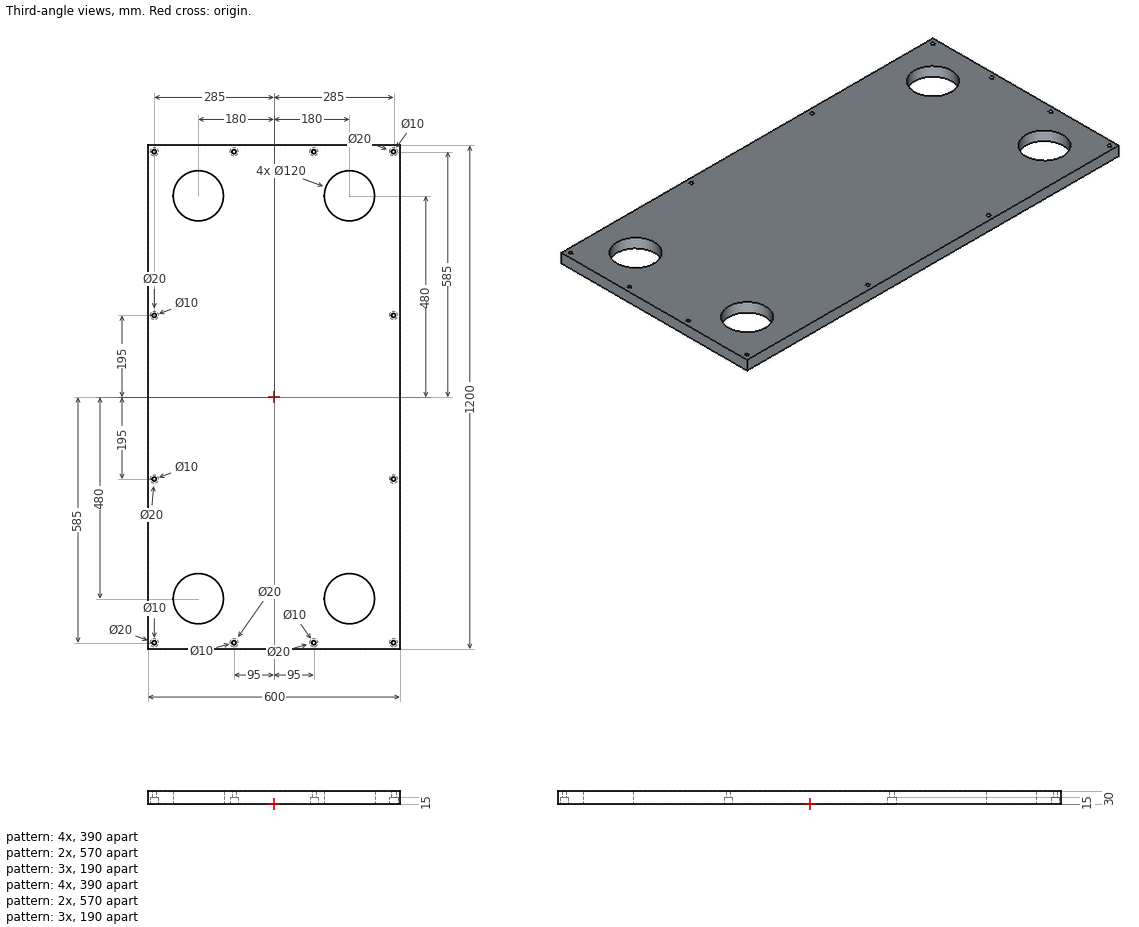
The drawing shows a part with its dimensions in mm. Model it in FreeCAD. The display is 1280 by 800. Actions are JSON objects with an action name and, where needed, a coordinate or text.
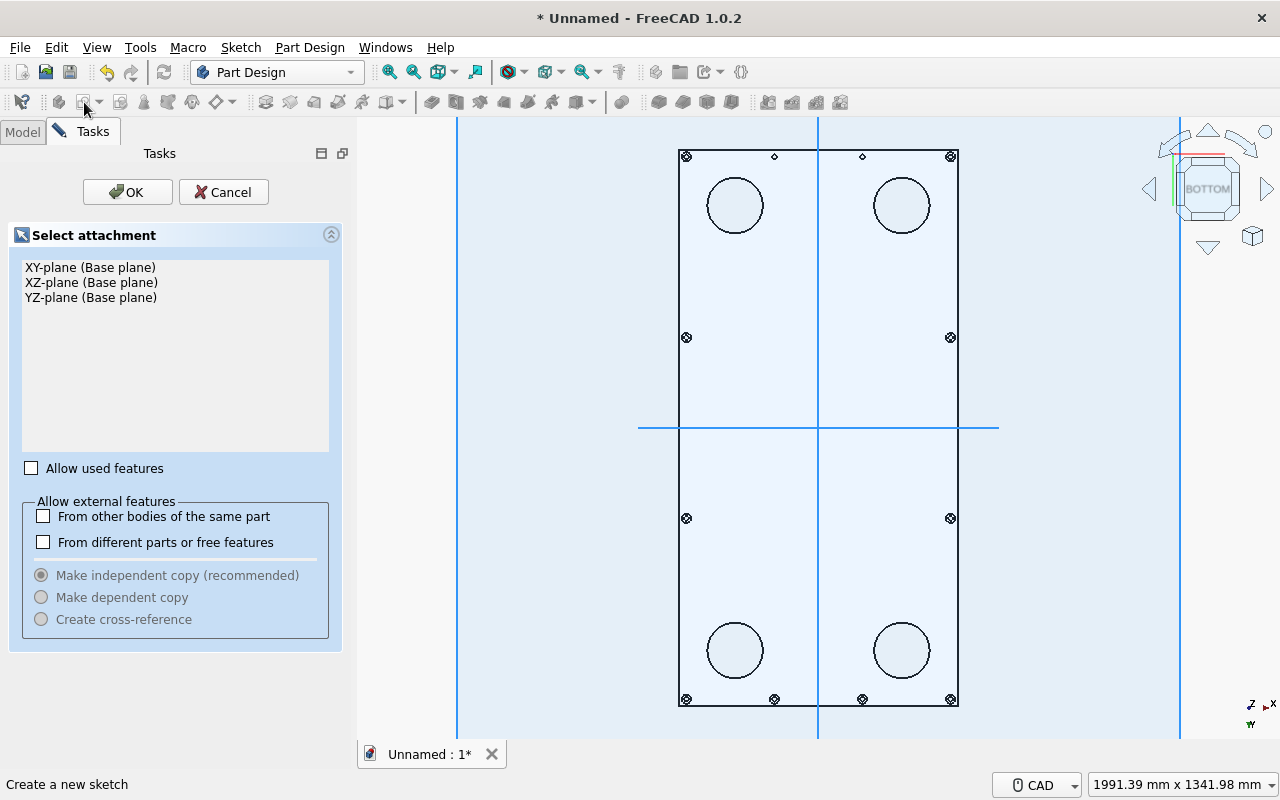
{"action": "left_click", "coordinate": [82, 268]}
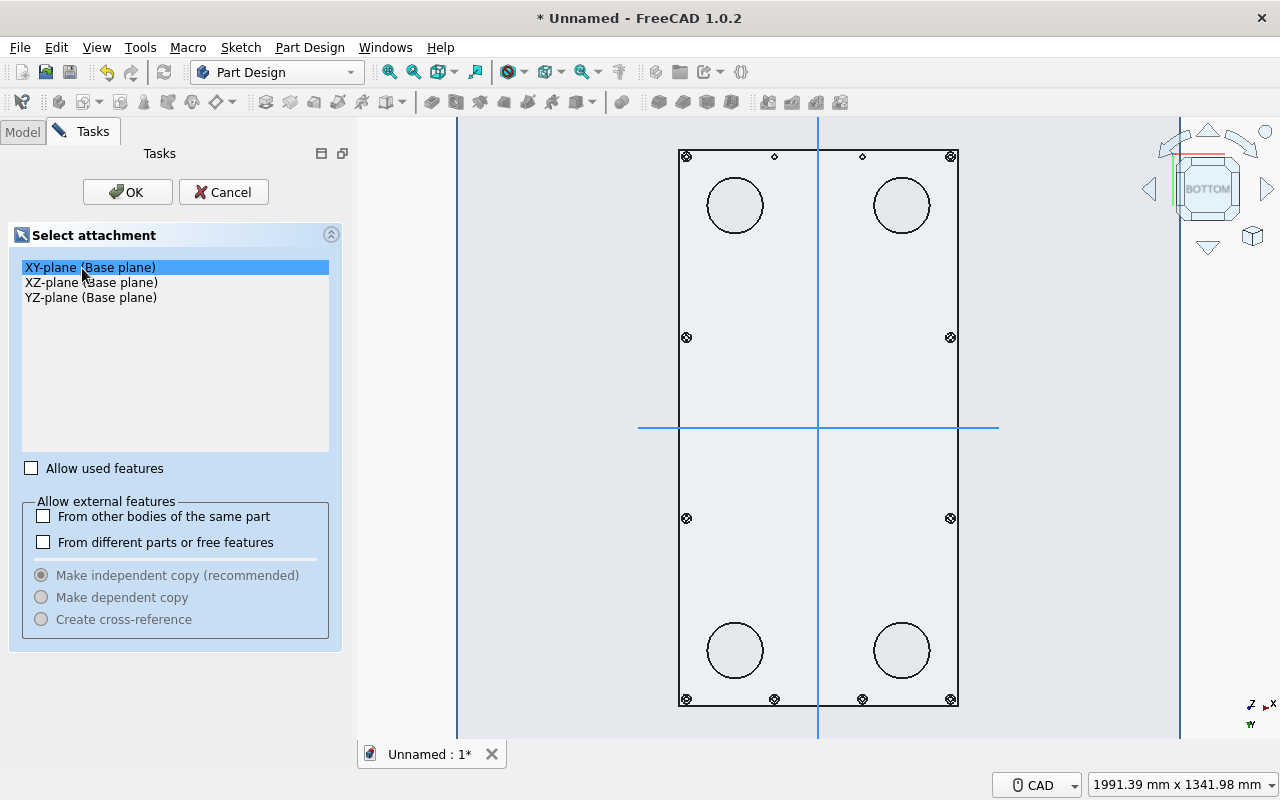
{"action": "left_click", "coordinate": [128, 192]}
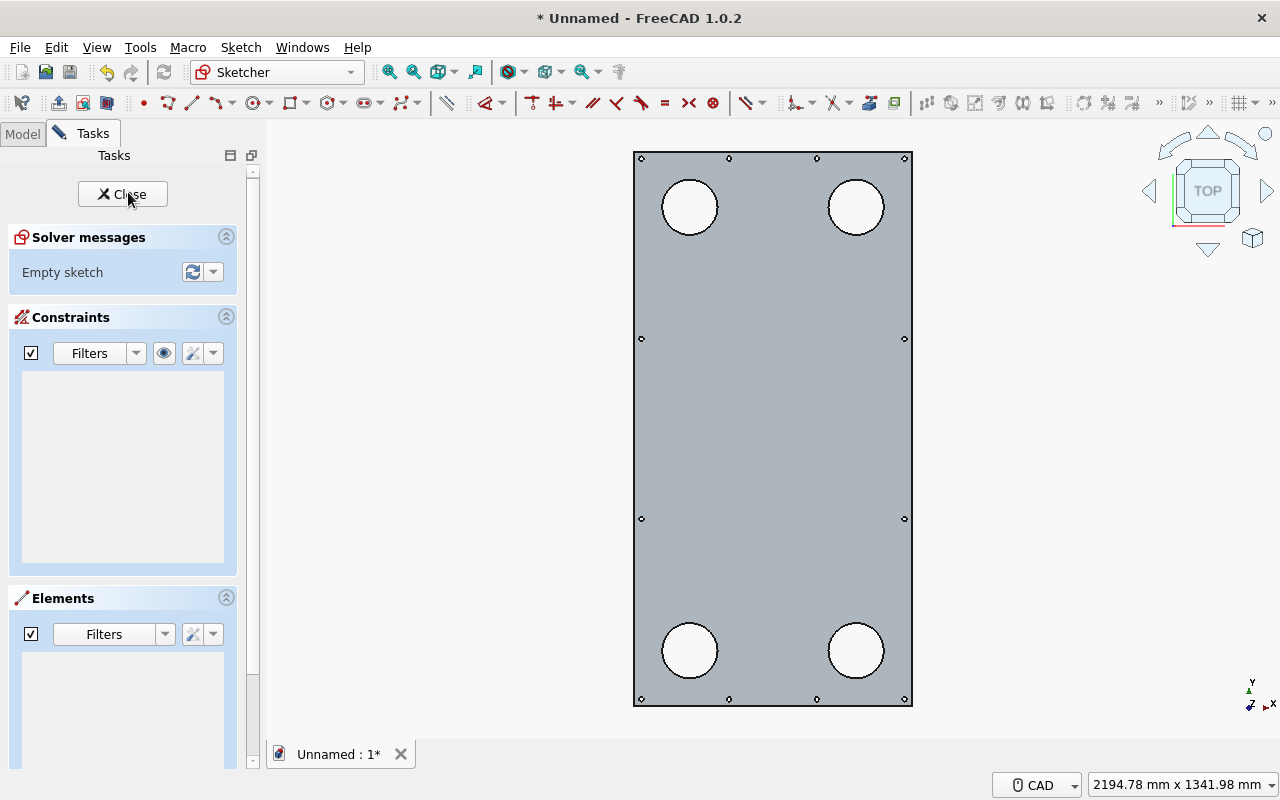
{"action": "left_click", "coordinate": [108, 104]}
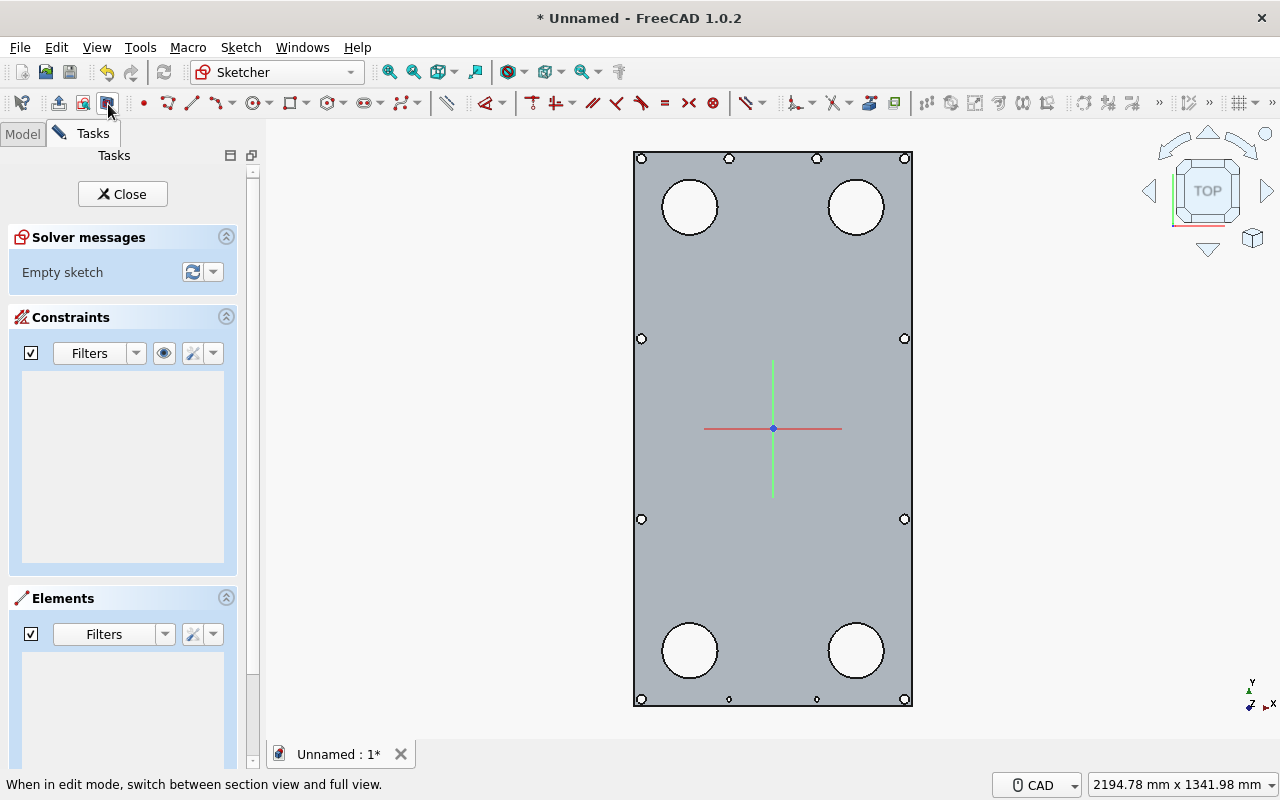
{"action": "scroll", "coordinate": [823, 711], "scroll_direction": "up", "scroll_amount": 15}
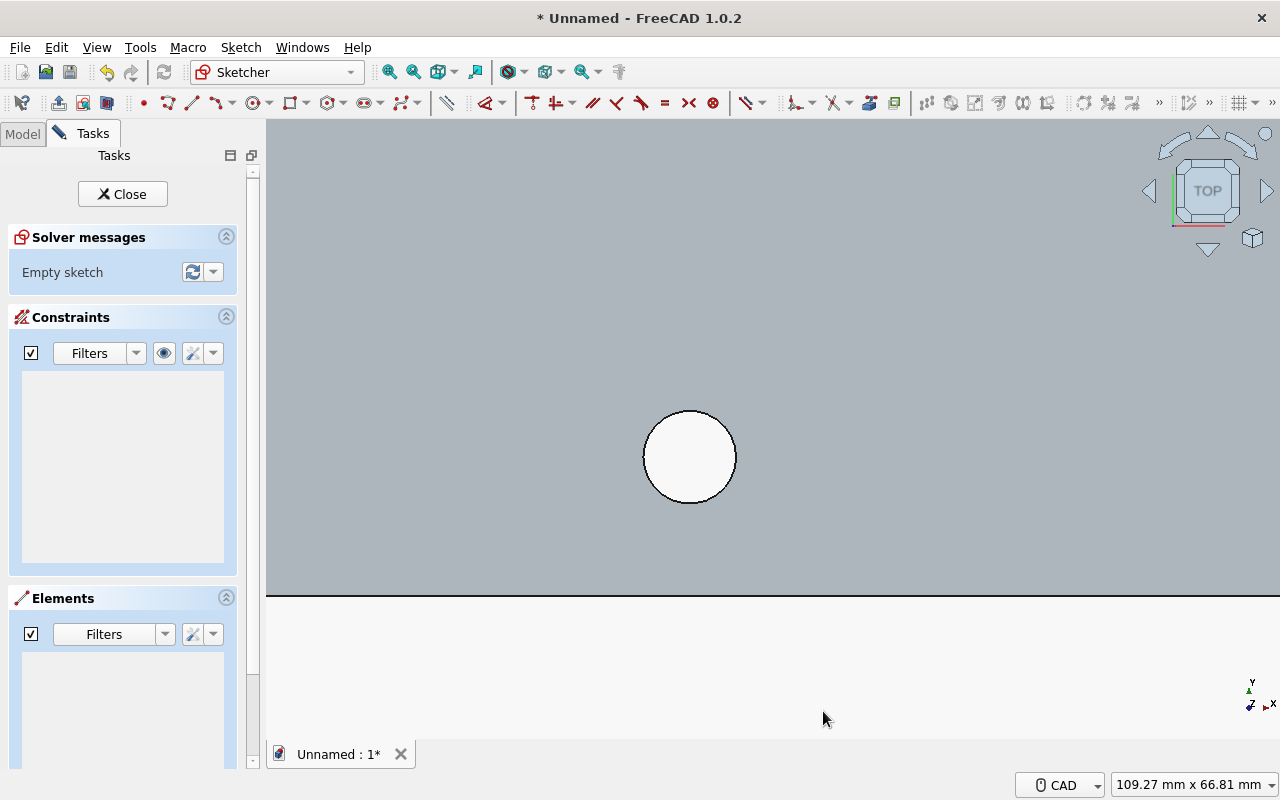
{"action": "scroll", "coordinate": [678, 480], "scroll_direction": "up", "scroll_amount": 4}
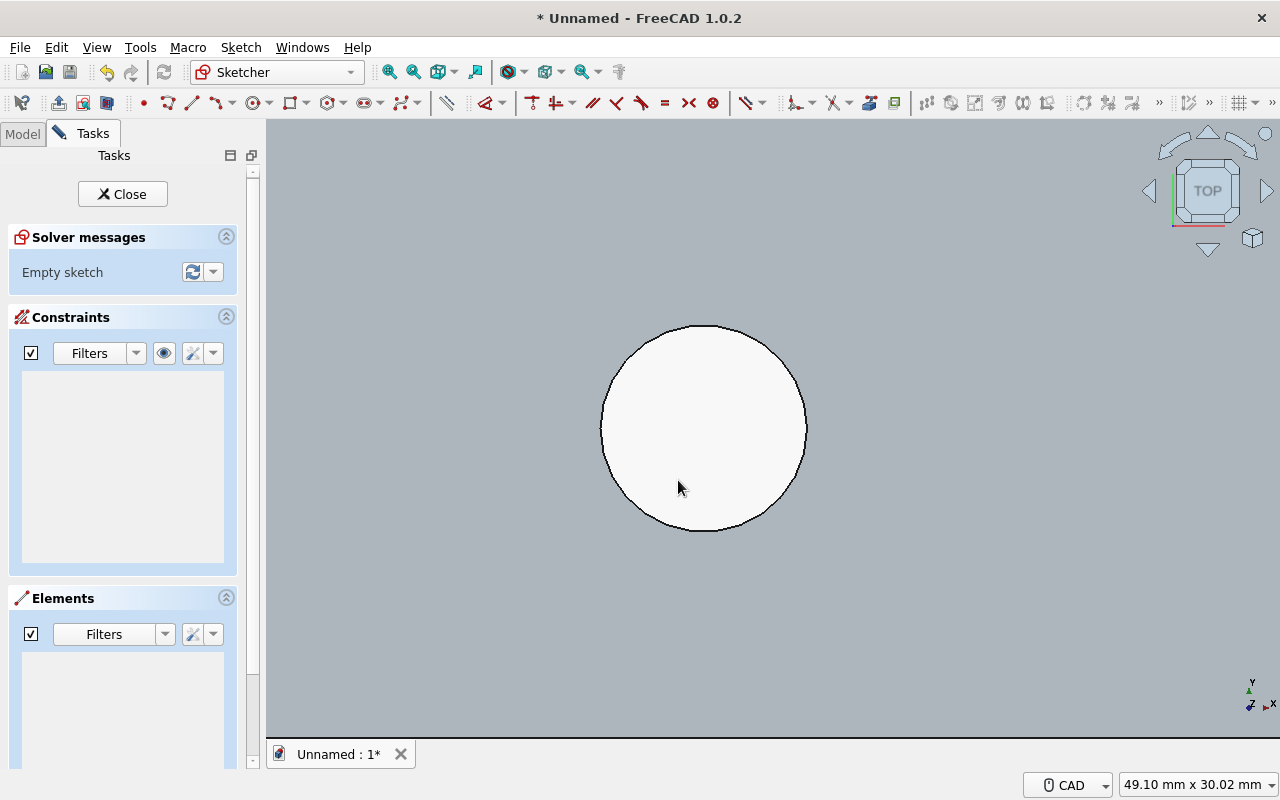
{"action": "left_click", "coordinate": [254, 104]}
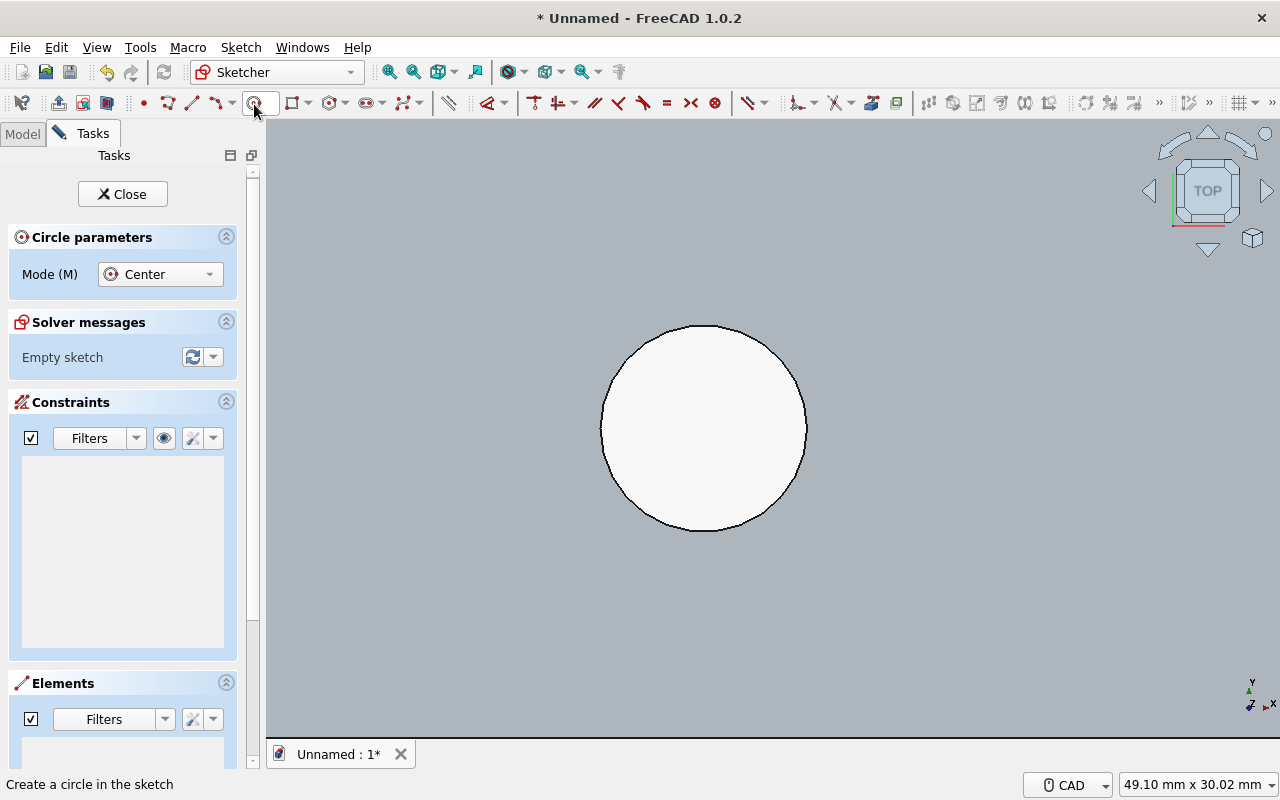
{"action": "left_click", "coordinate": [704, 429]}
{"action": "mouse_move", "coordinate": [850, 283]}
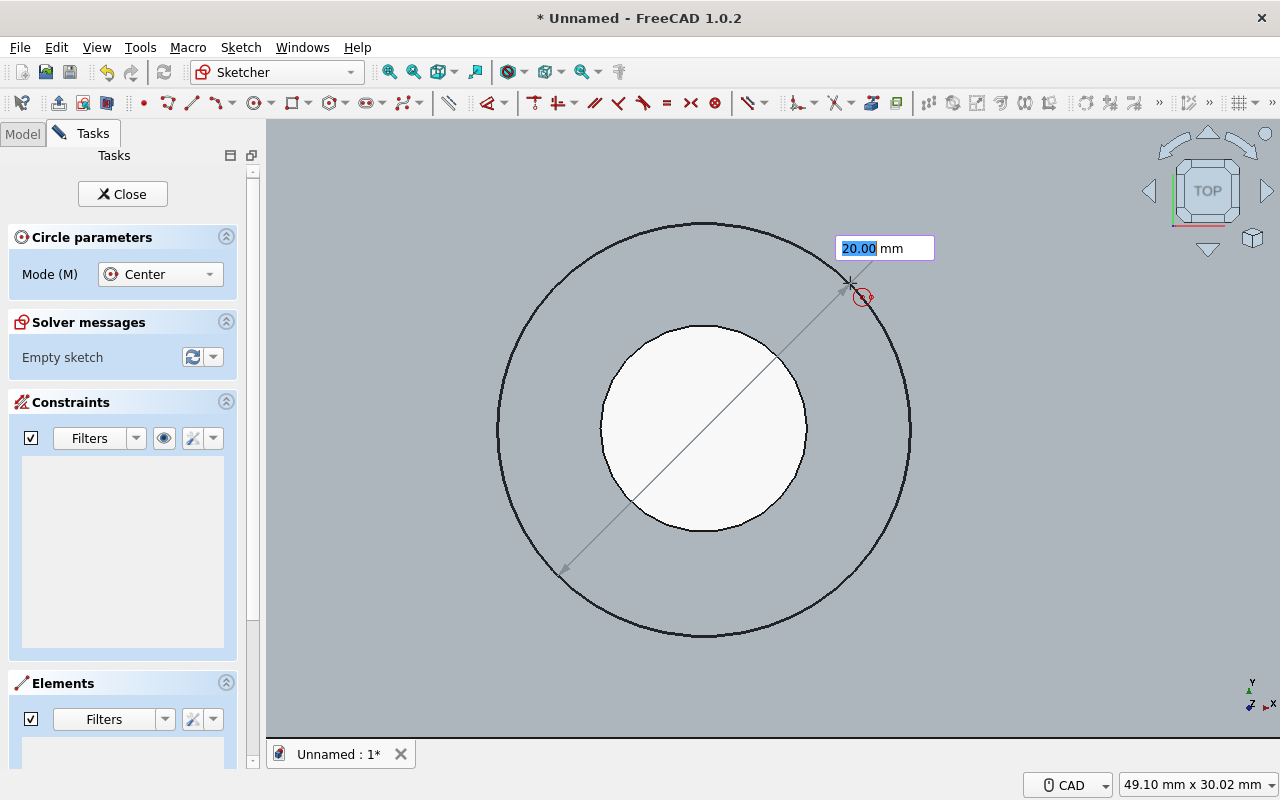
{"action": "type", "text": "20"}
{"action": "key", "text": "Return"}
{"action": "key", "text": "Escape"}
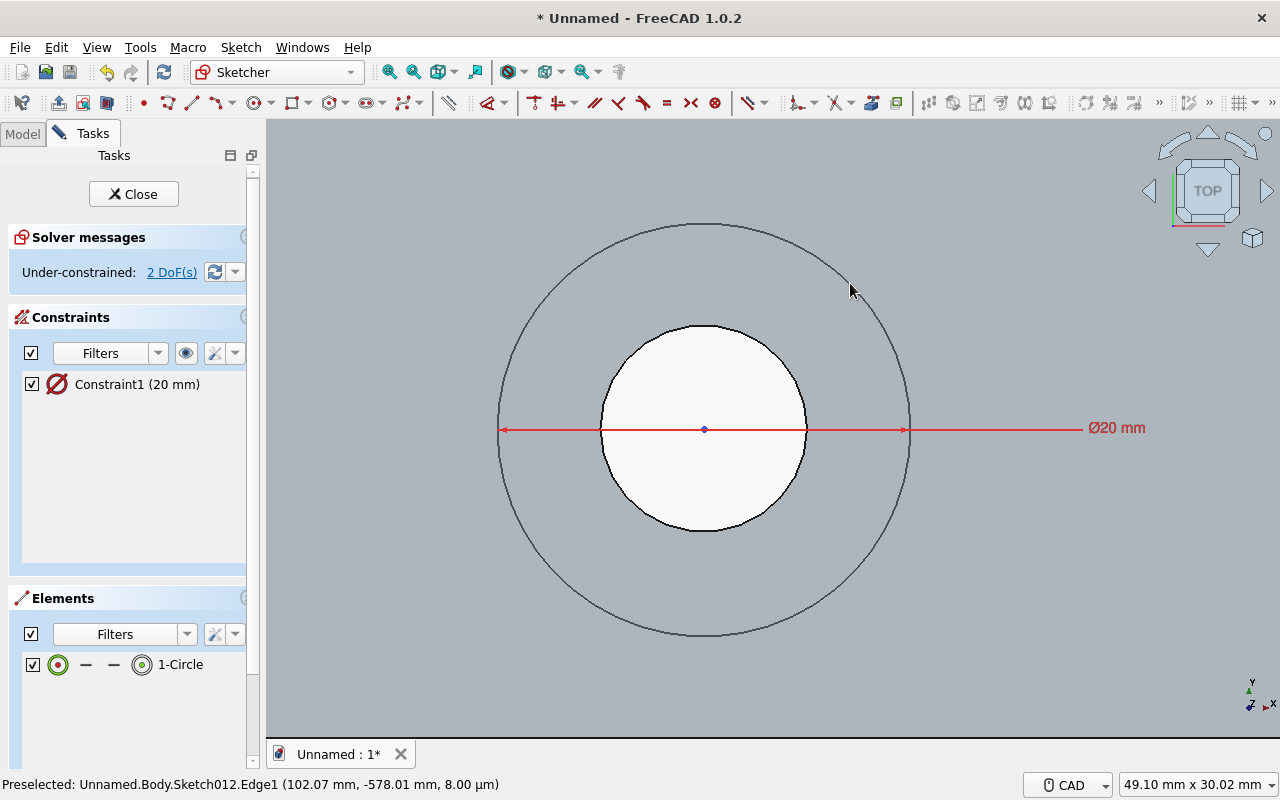
{"action": "left_click", "coordinate": [488, 104]}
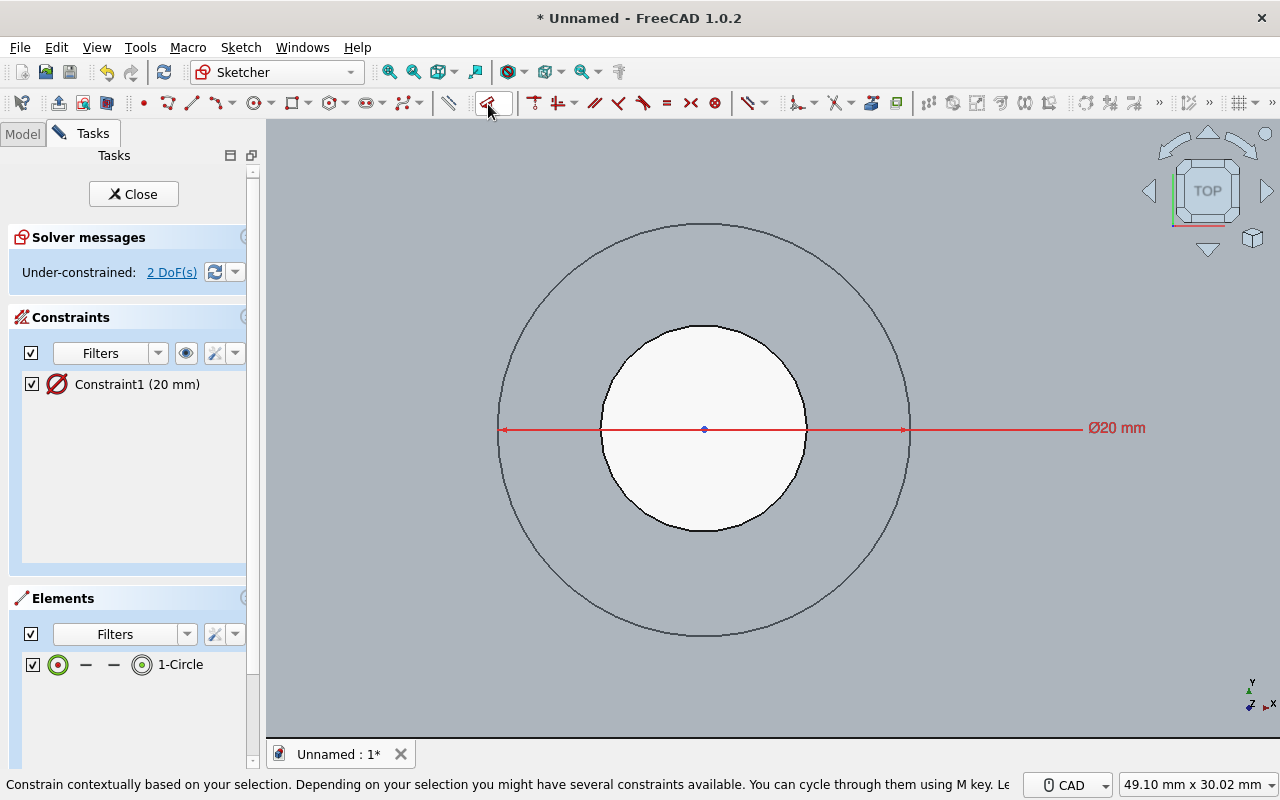
{"action": "left_click", "coordinate": [704, 430]}
{"action": "left_click", "coordinate": [405, 464]}